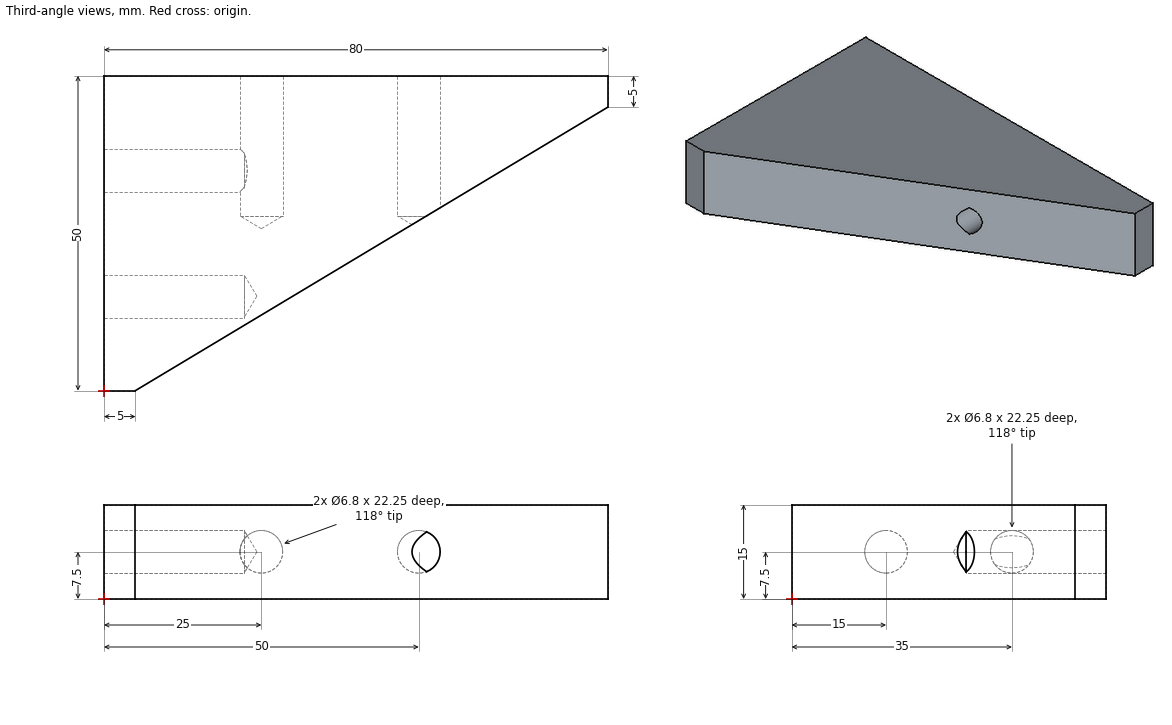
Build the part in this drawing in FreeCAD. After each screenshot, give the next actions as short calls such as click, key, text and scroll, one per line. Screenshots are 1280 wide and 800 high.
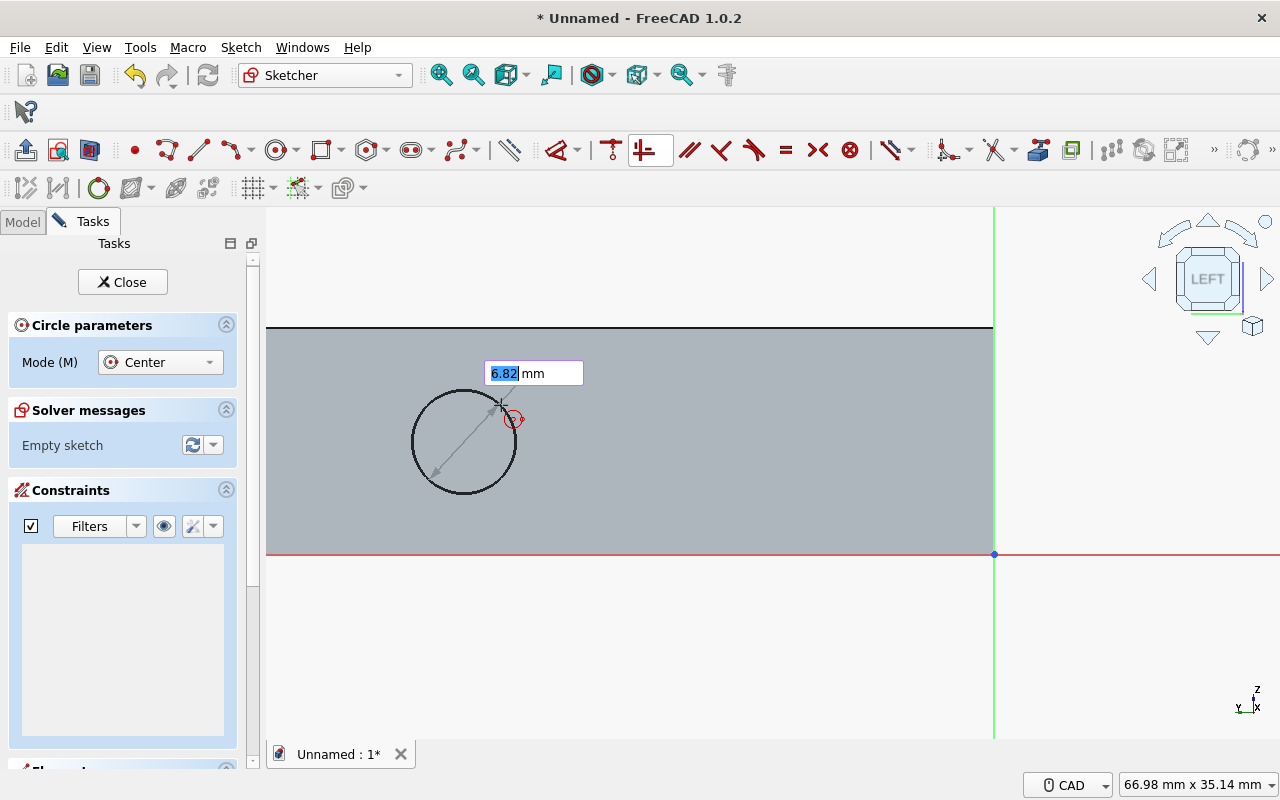
text(6.8)
key(Return)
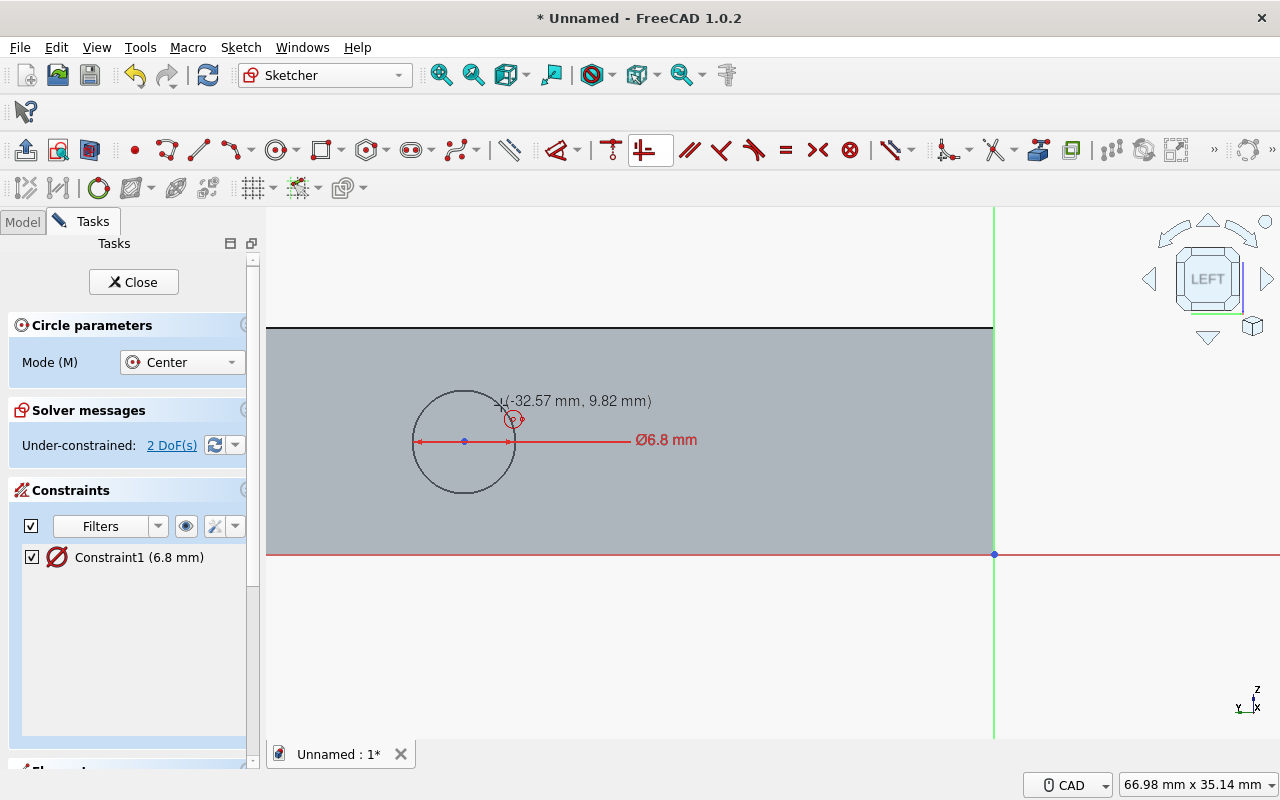
click(767, 441)
move(803, 405)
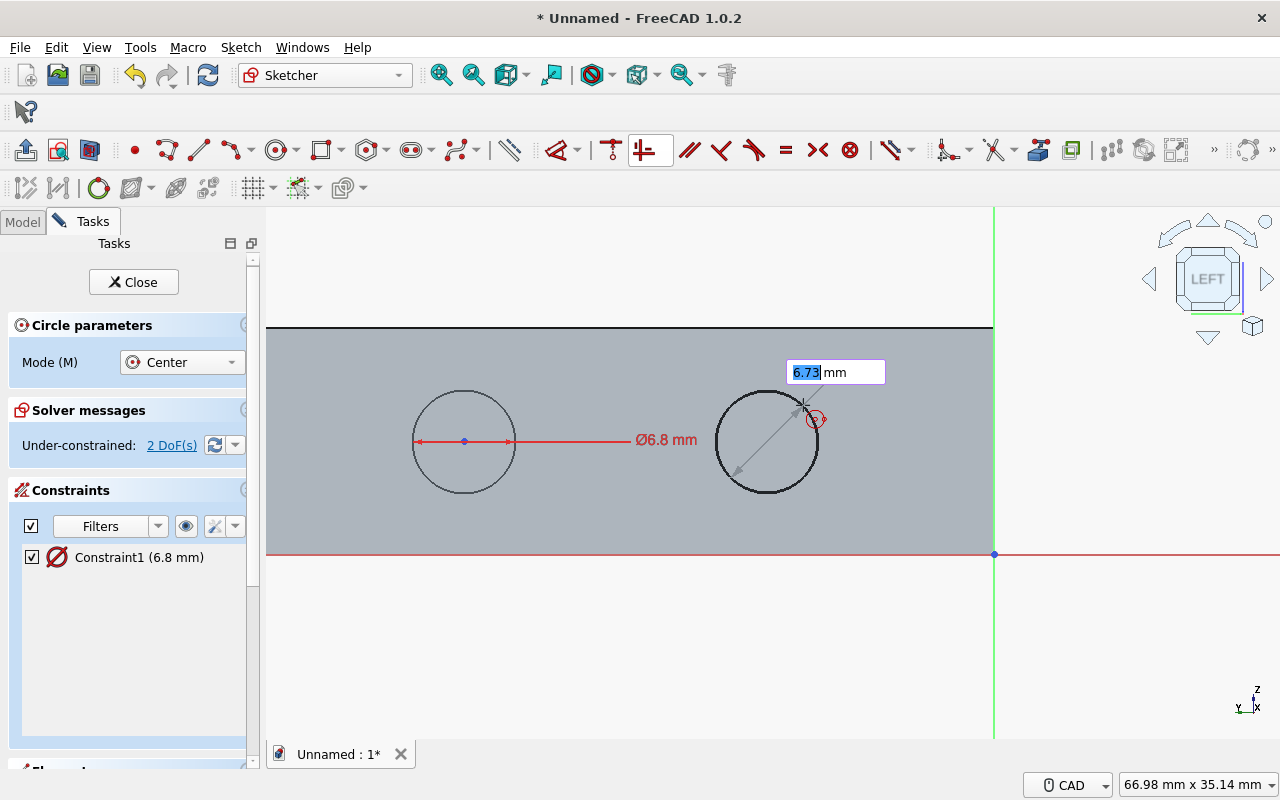
text(6.8)
key(Return)
key(Escape)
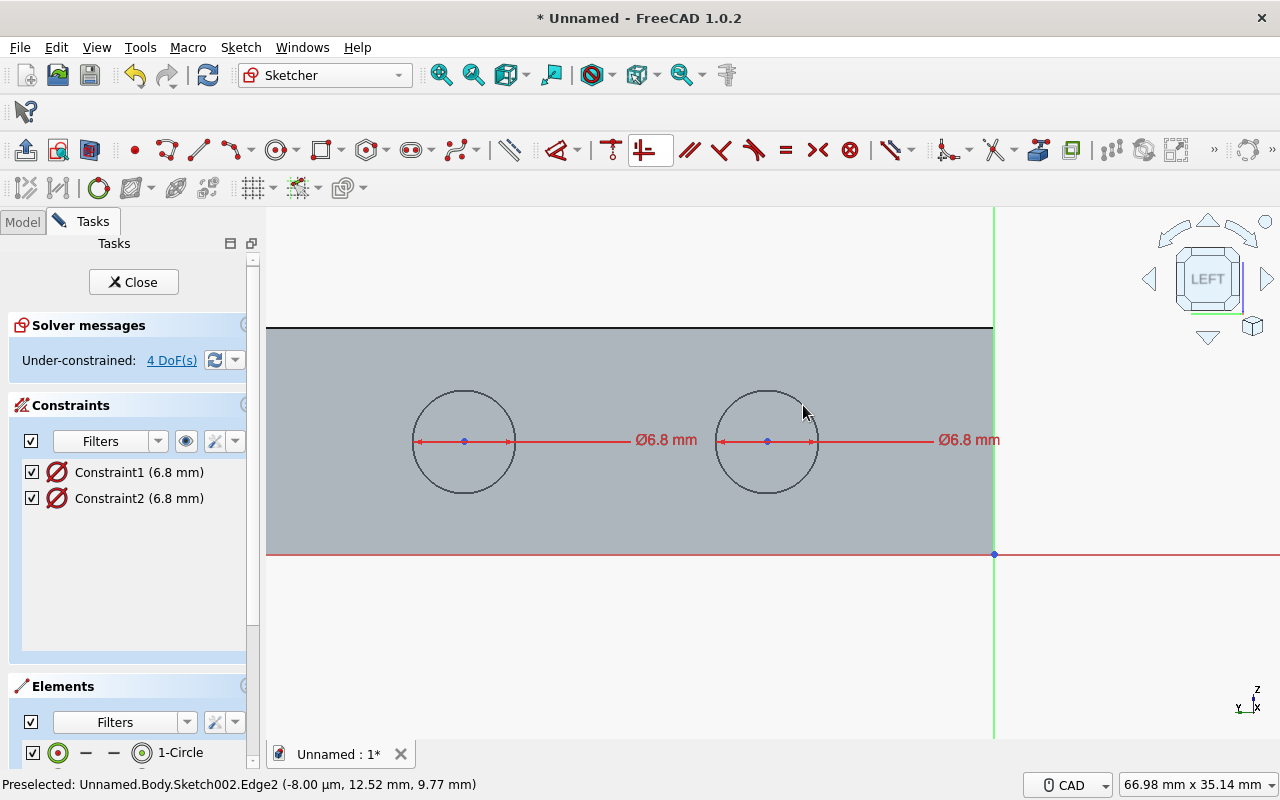
key(d)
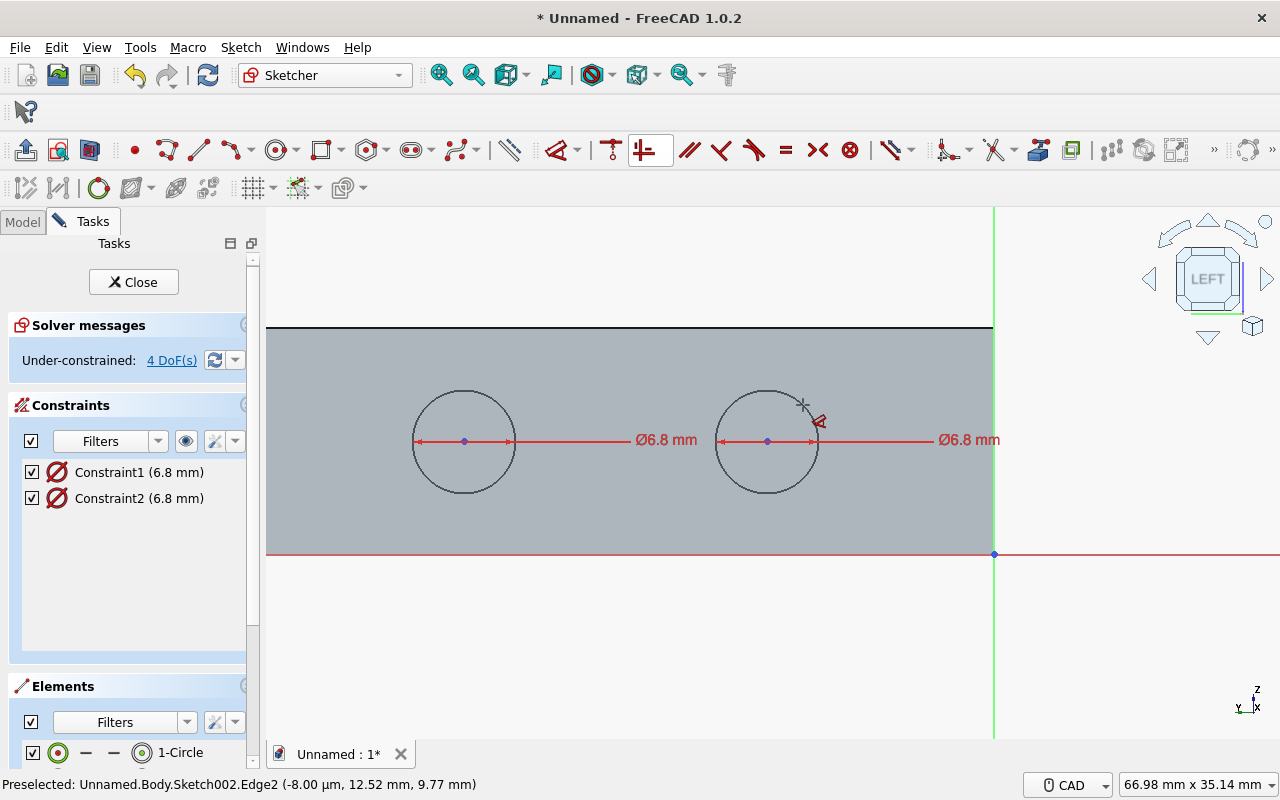
click(464, 442)
click(729, 589)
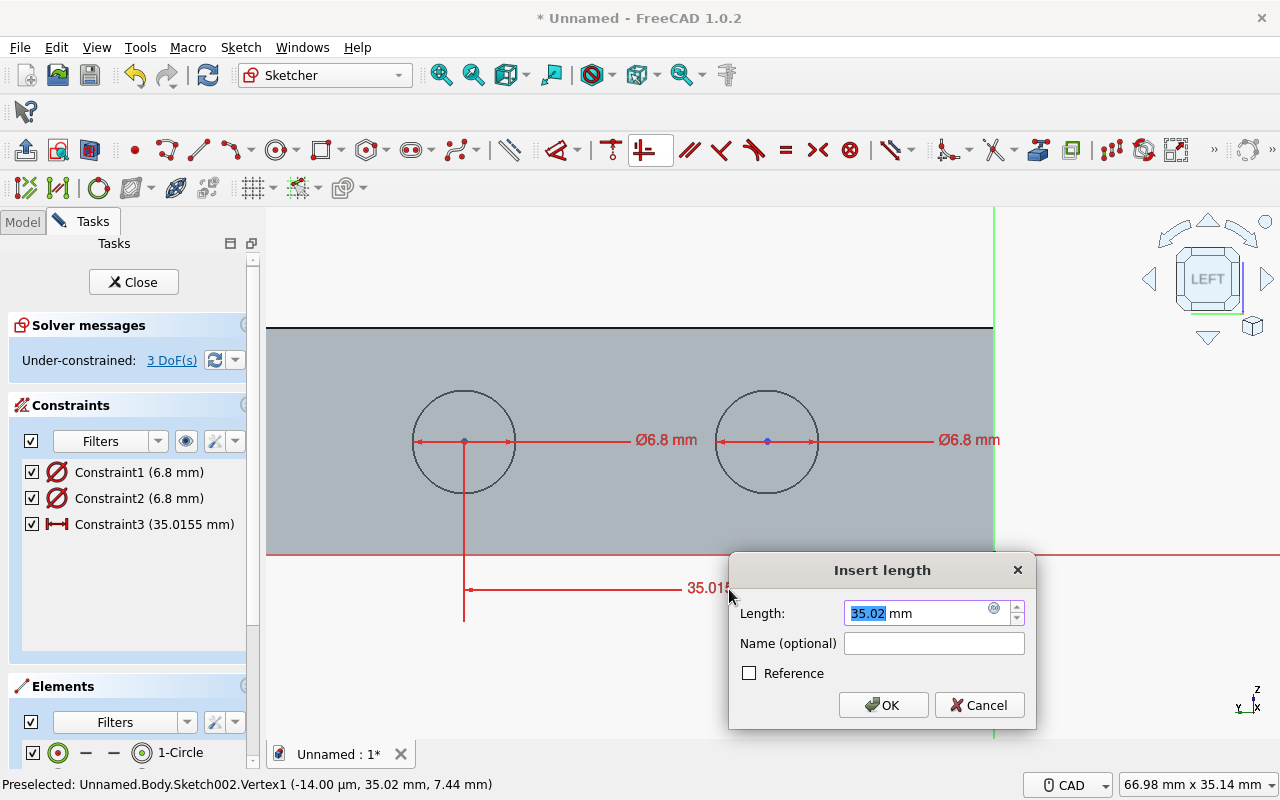
text(35)
key(Return)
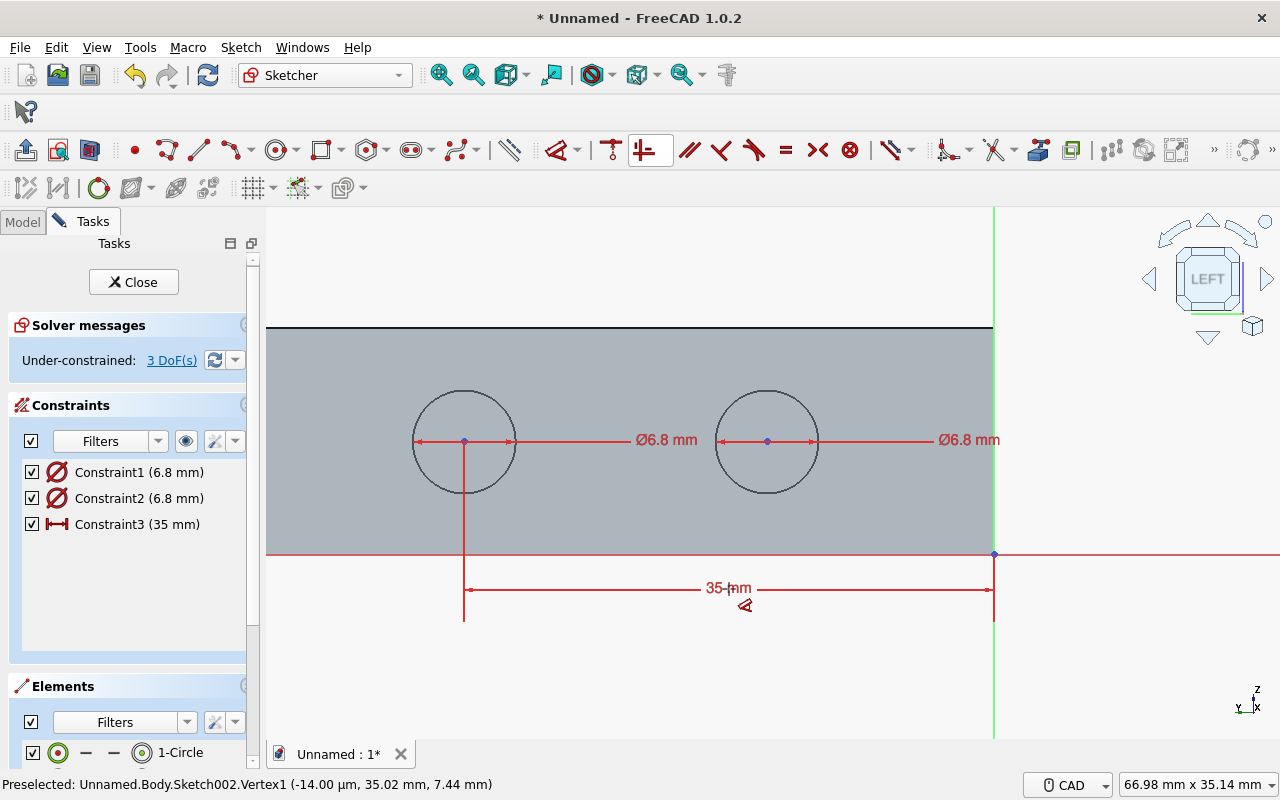
click(767, 442)
click(881, 589)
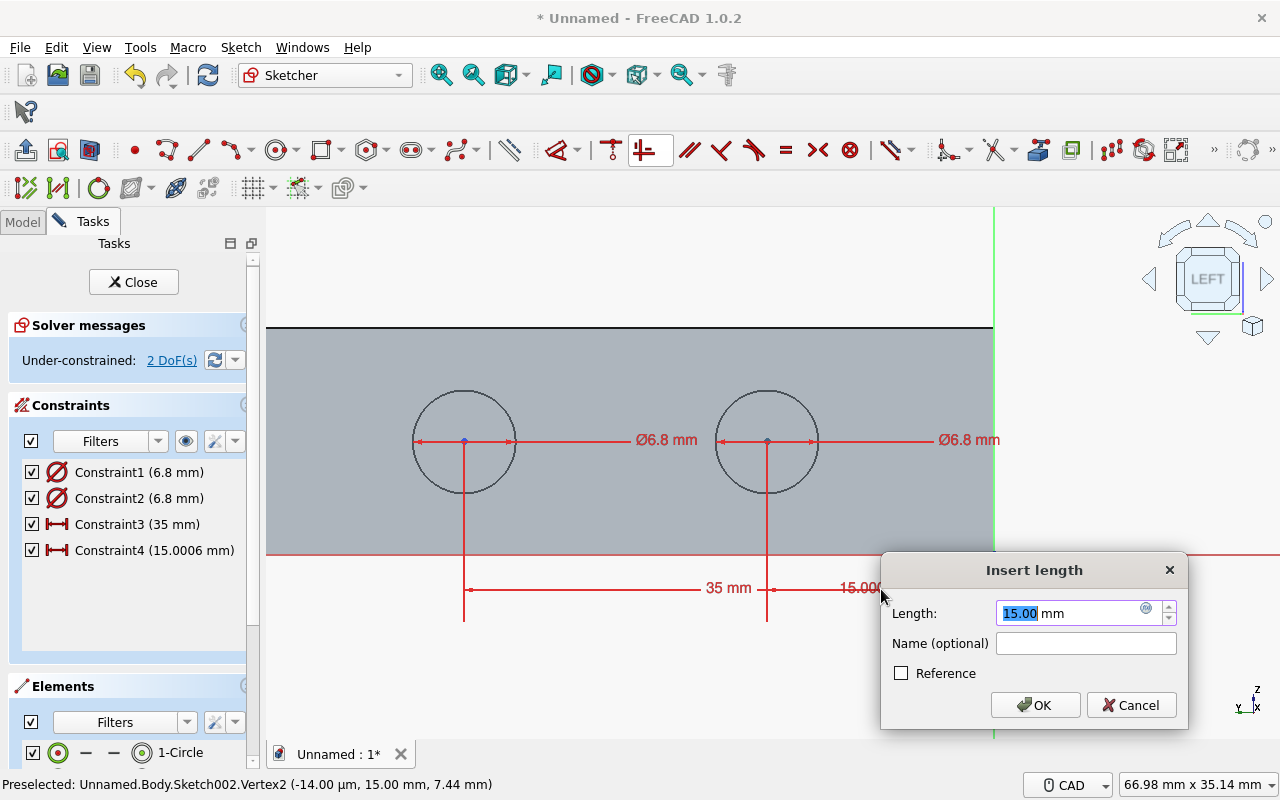
text(15)
key(Return)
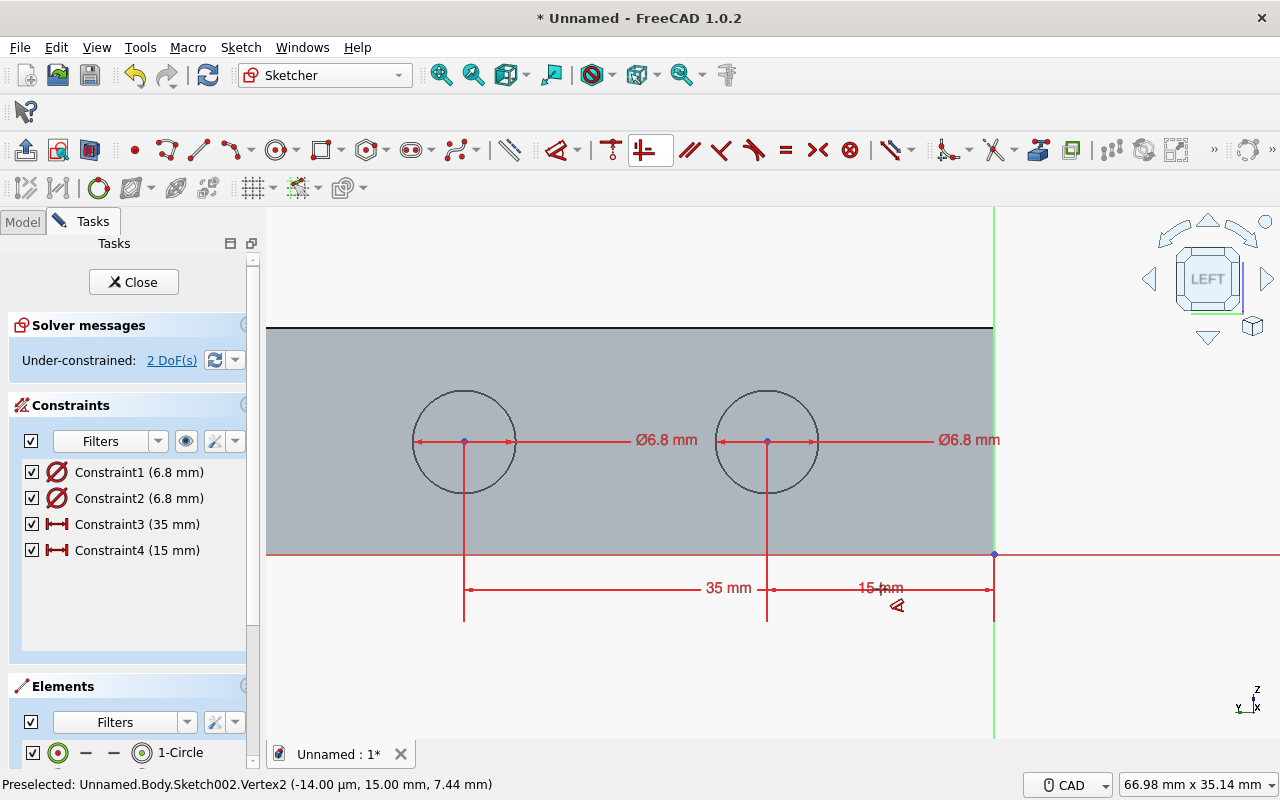
click(464, 442)
click(1028, 498)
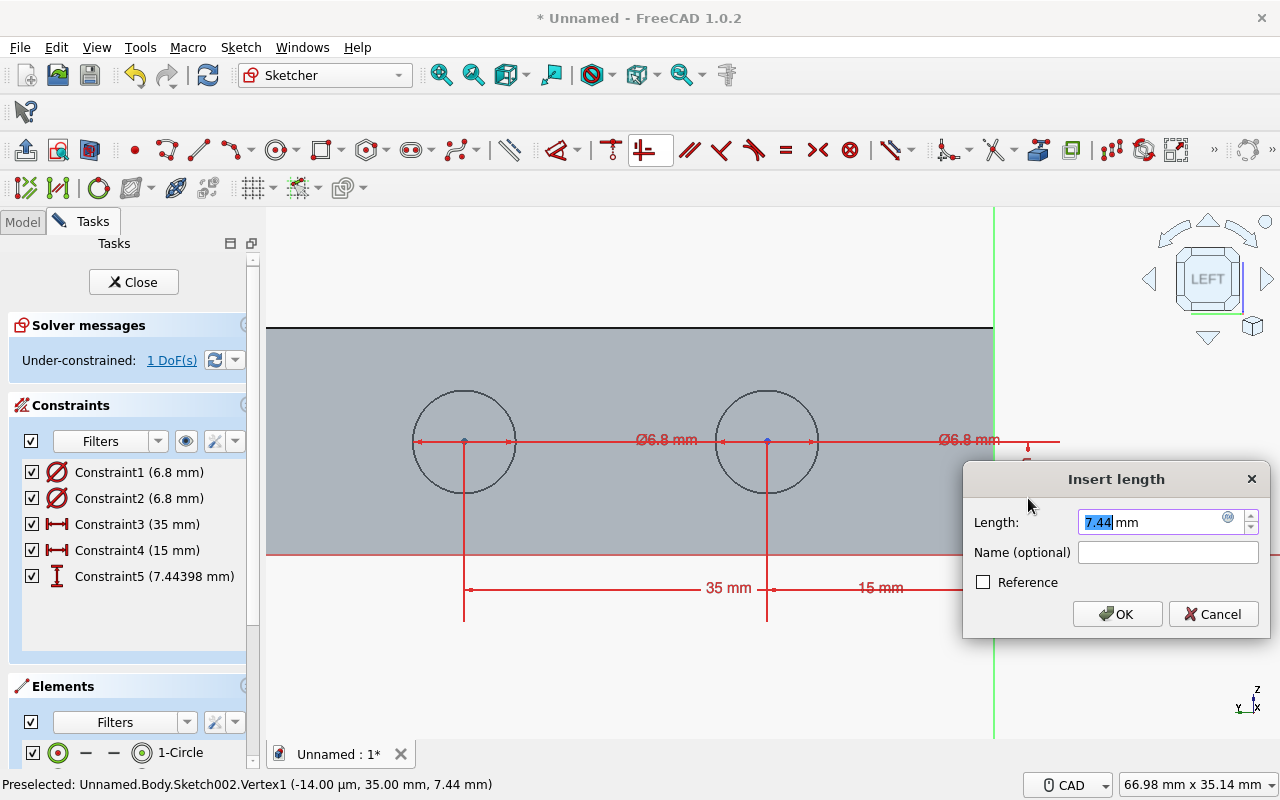
text(7.5)
key(Return)